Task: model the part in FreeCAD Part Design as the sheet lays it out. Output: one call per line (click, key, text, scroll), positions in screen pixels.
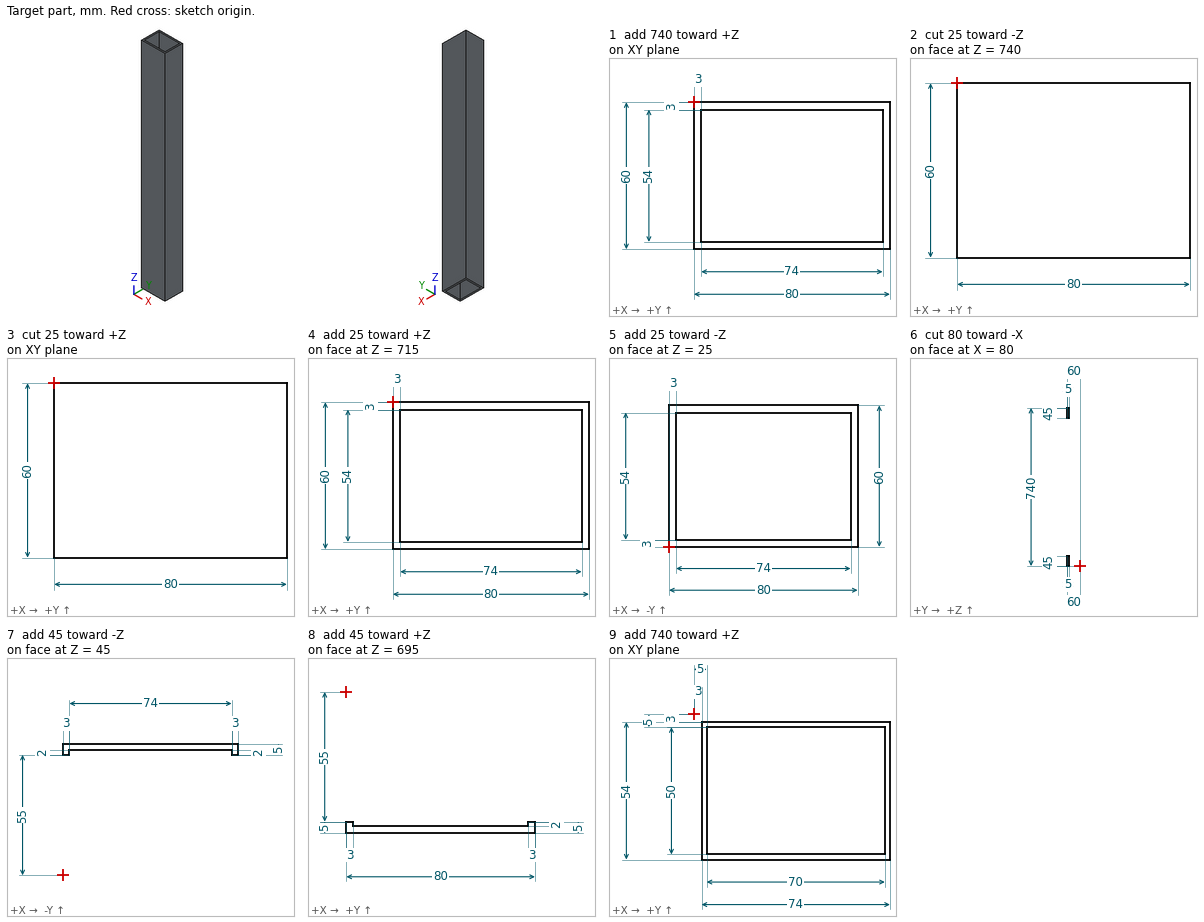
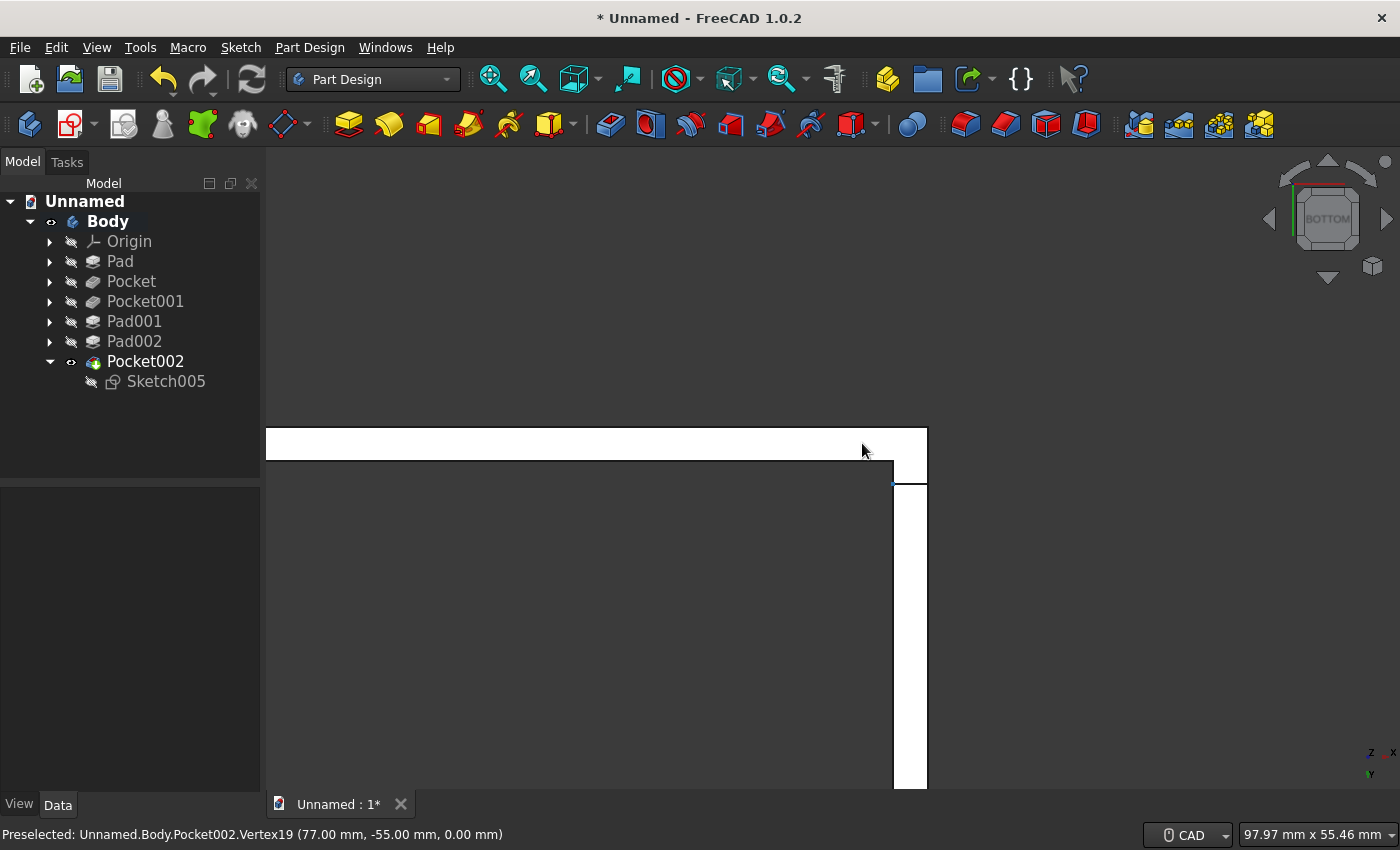
click(862, 446)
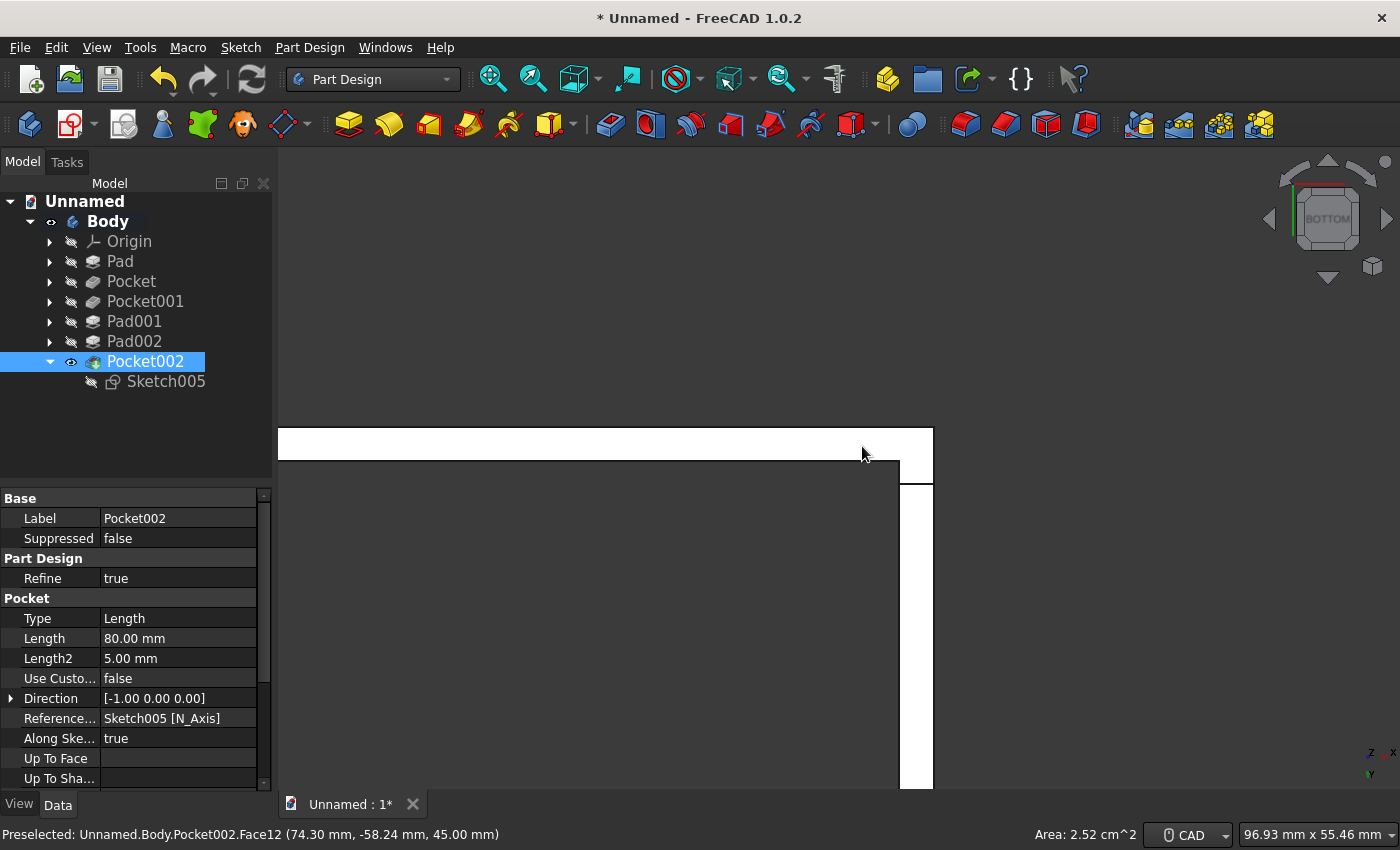
click(70, 124)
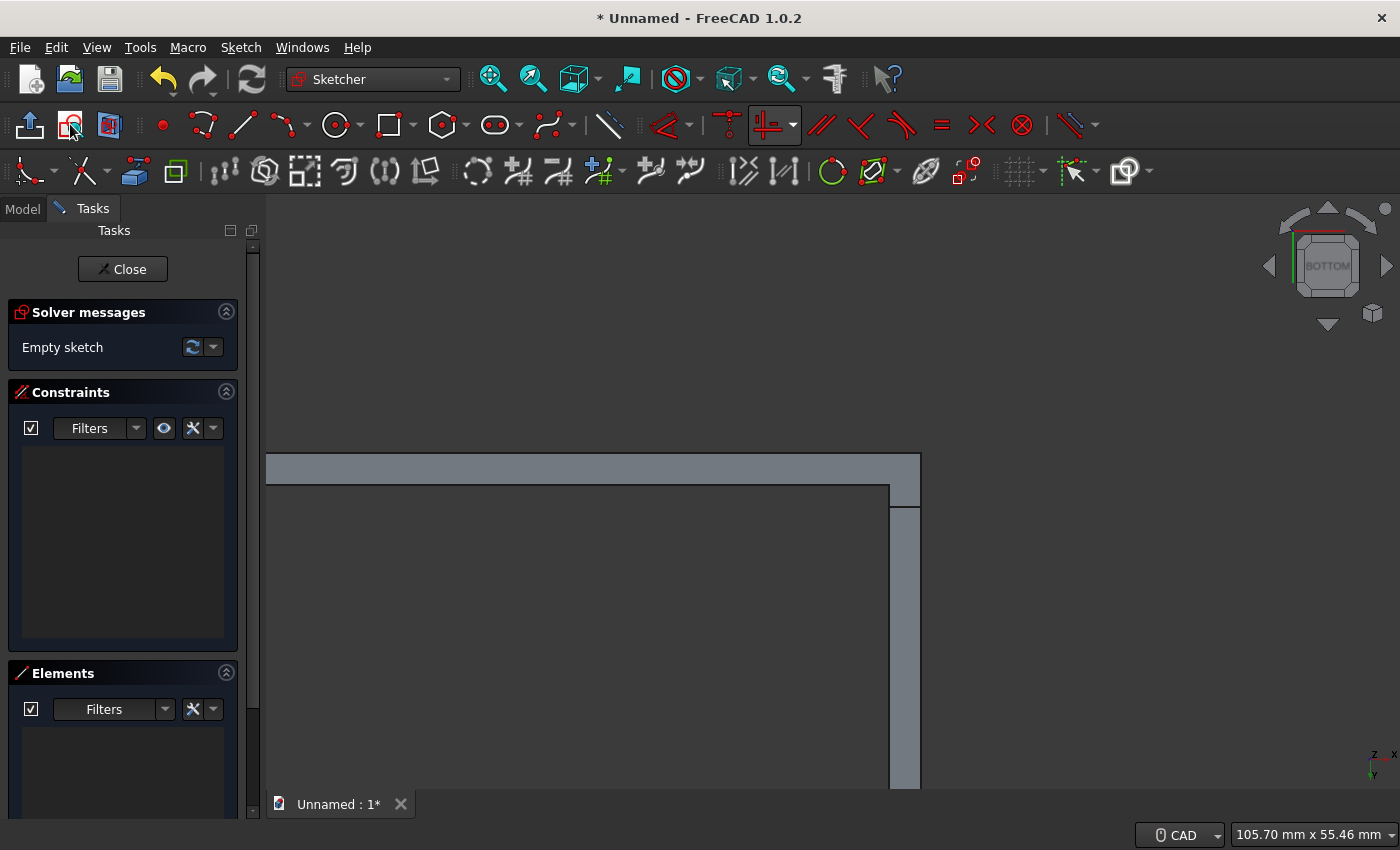
click(110, 126)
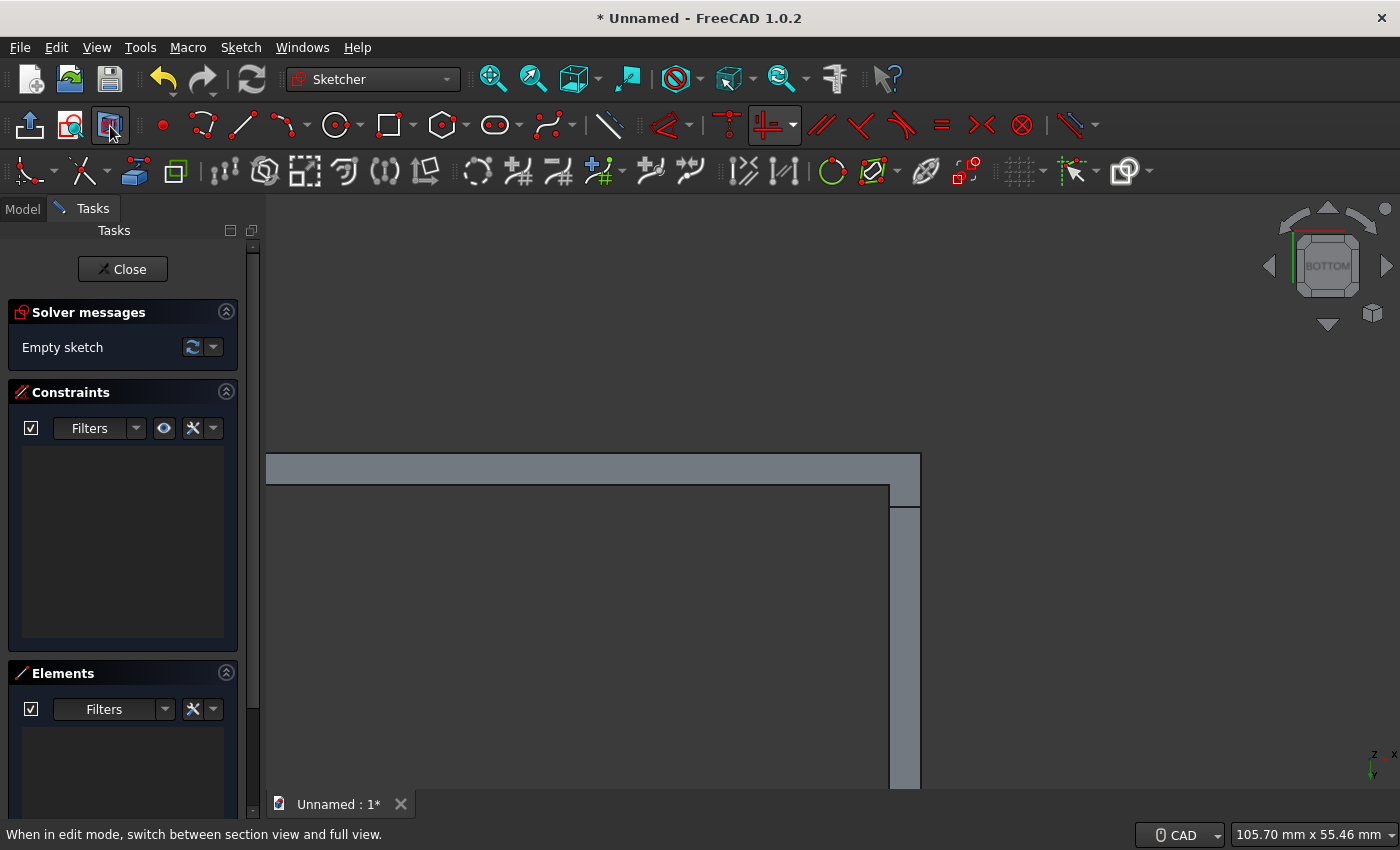
scroll(1096, 222, down, 3)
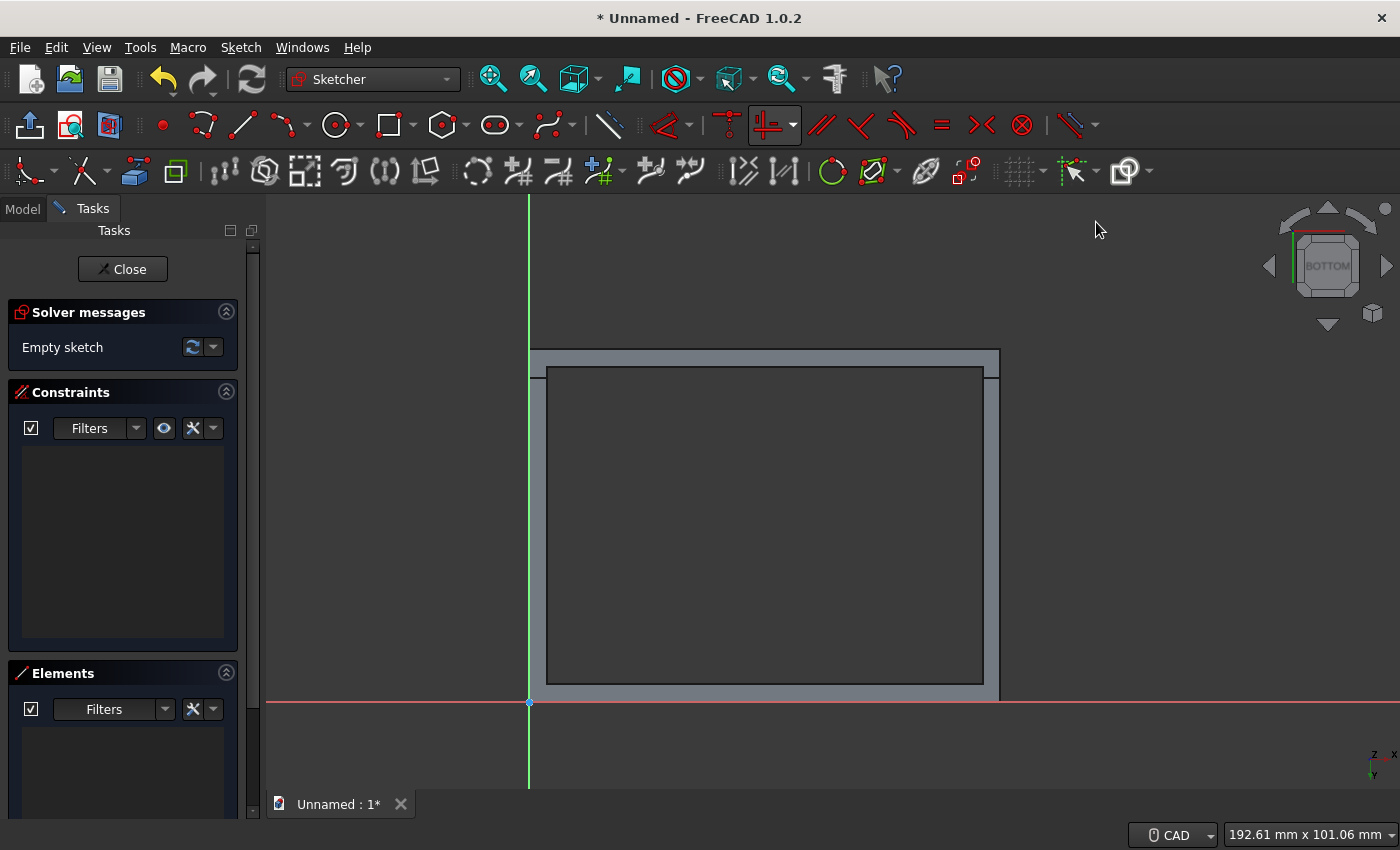
key(g)
key(m)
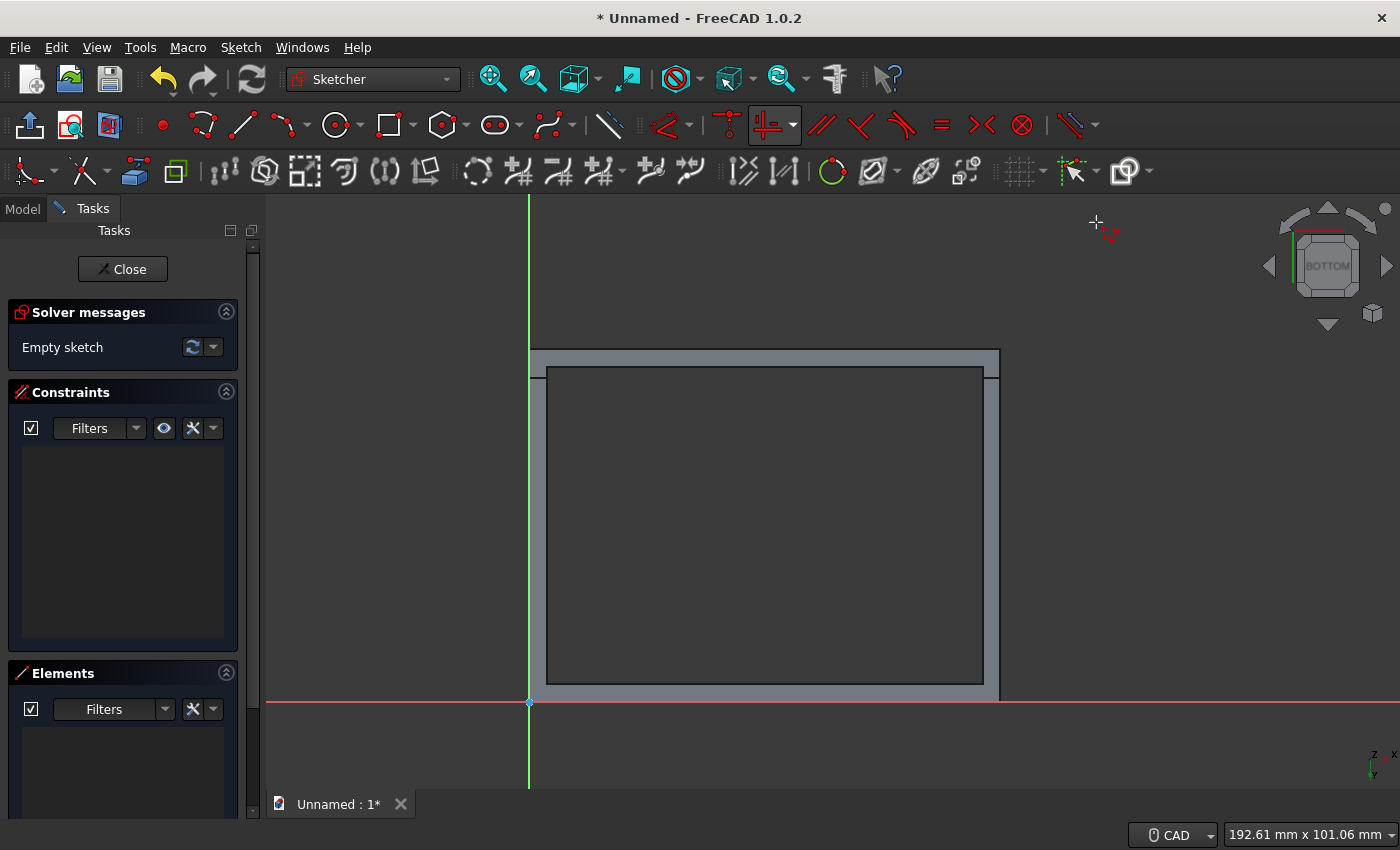
click(529, 378)
click(547, 378)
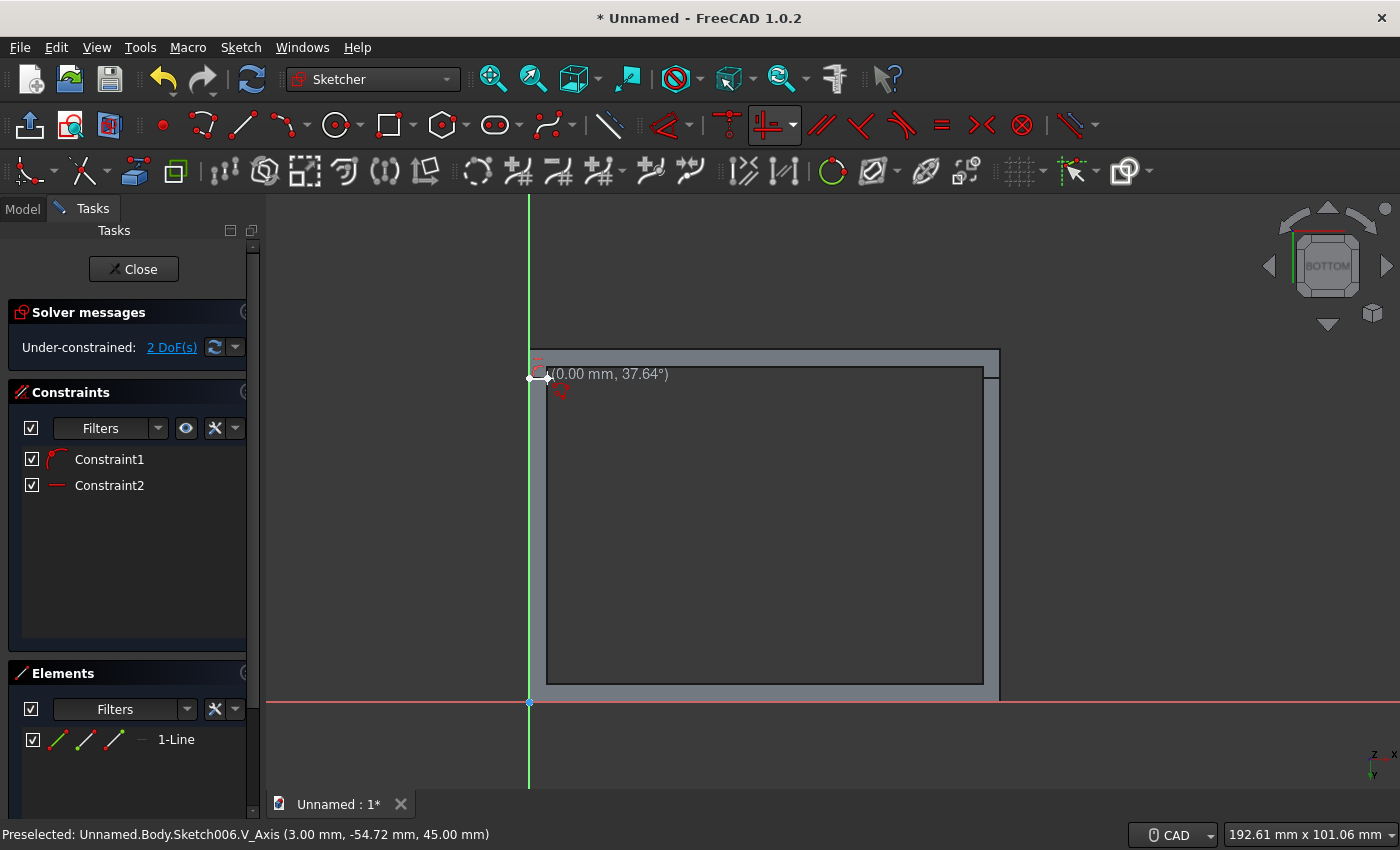
scroll(547, 367, up, 2)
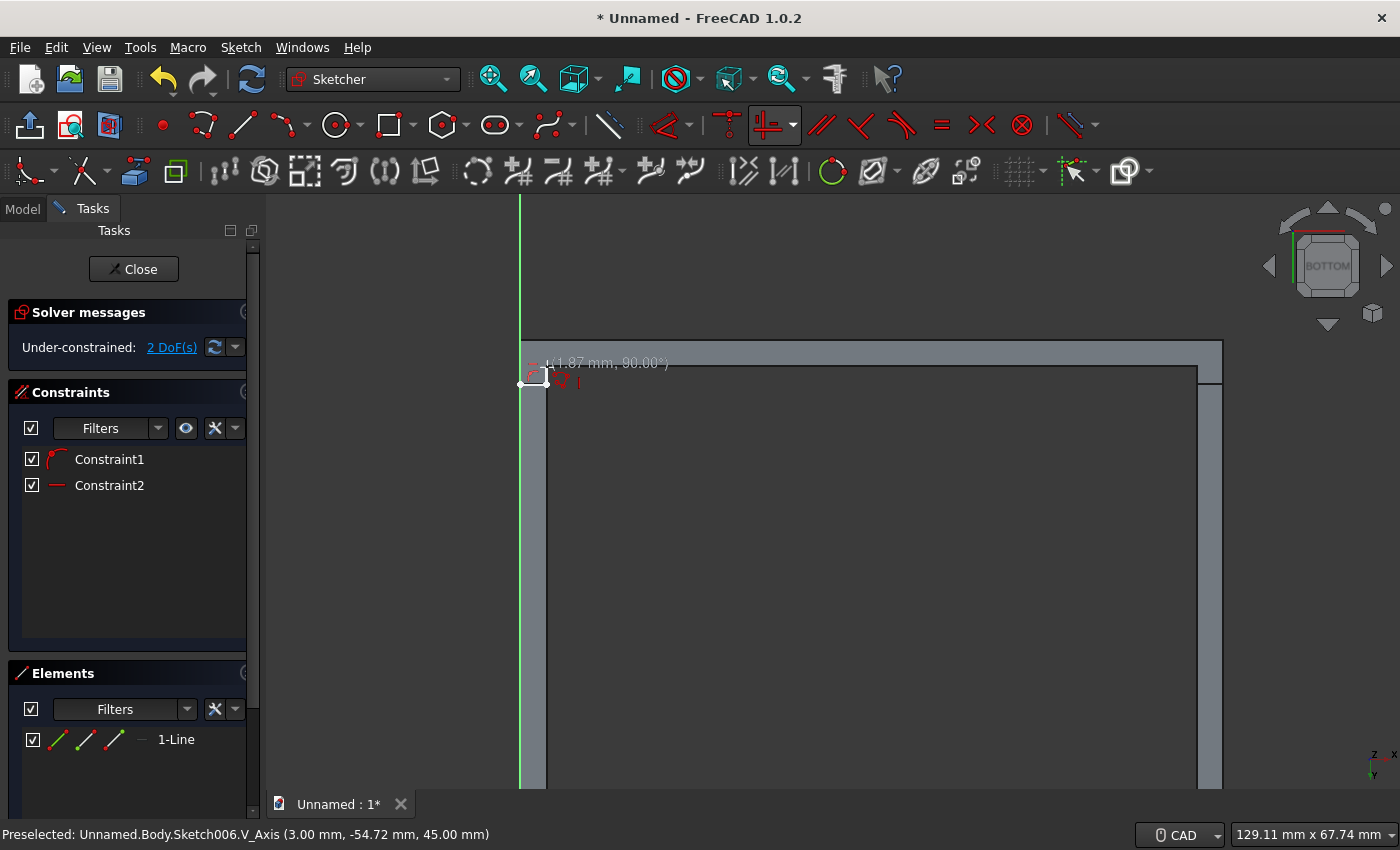
click(547, 366)
click(1197, 366)
click(1197, 384)
click(1223, 384)
click(1223, 340)
click(529, 340)
click(520, 385)
key(Escape)
key(Escape)